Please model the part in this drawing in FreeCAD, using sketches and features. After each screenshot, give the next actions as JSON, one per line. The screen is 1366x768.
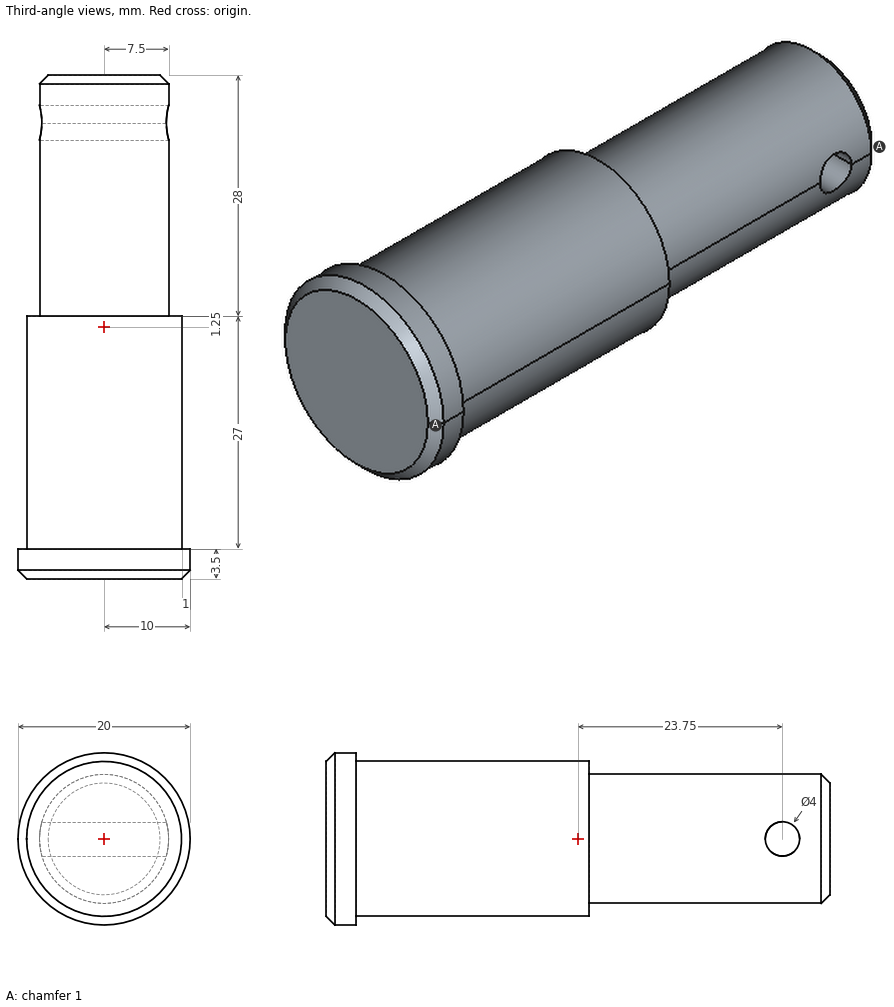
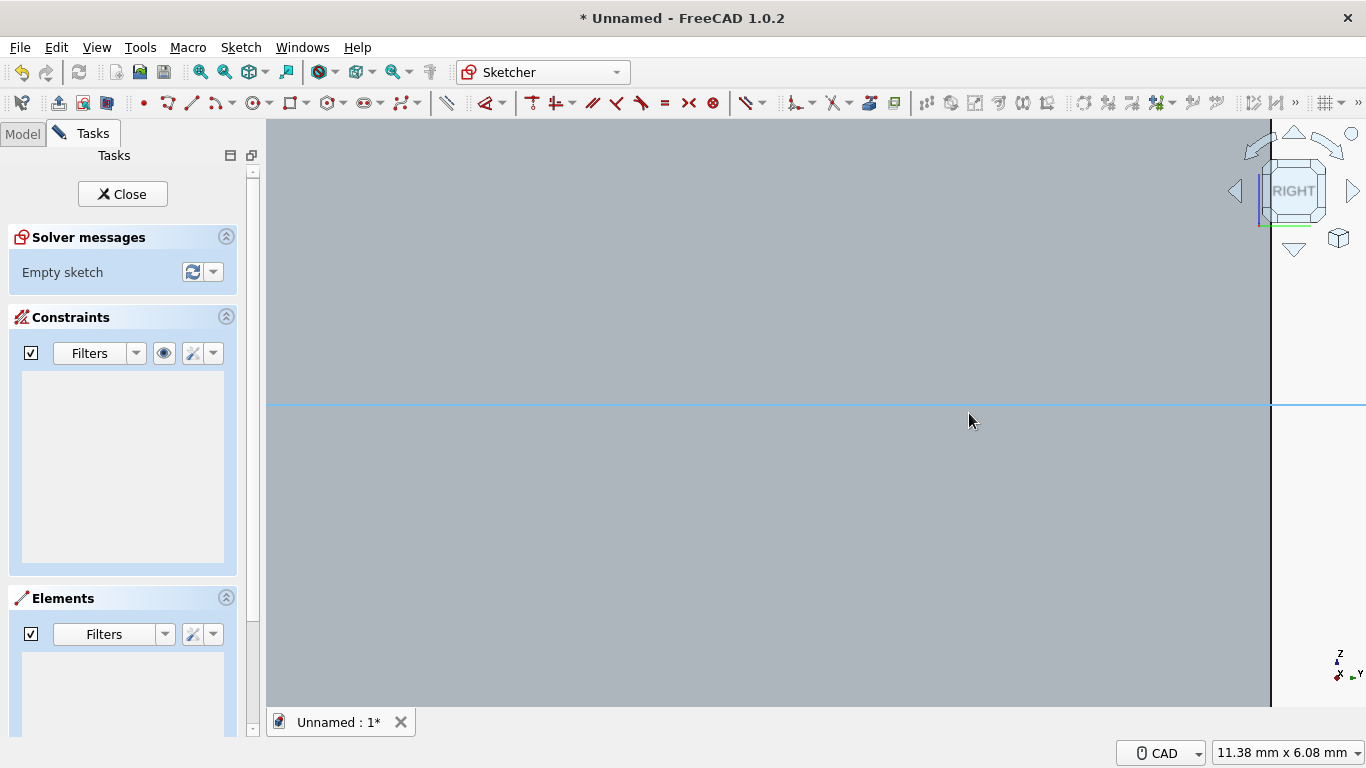
{"action": "left_click", "coordinate": [254, 104]}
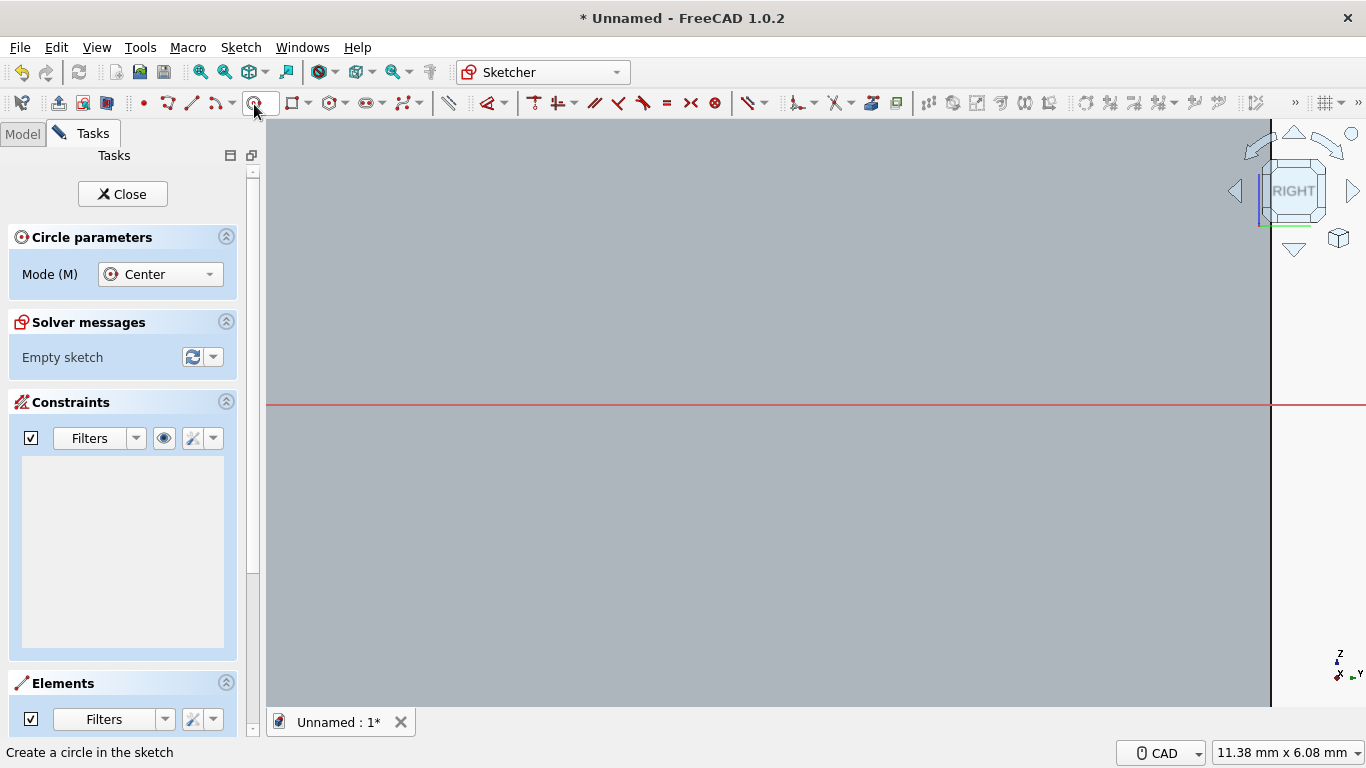
{"action": "left_click", "coordinate": [740, 405]}
{"action": "mouse_move", "coordinate": [876, 269]}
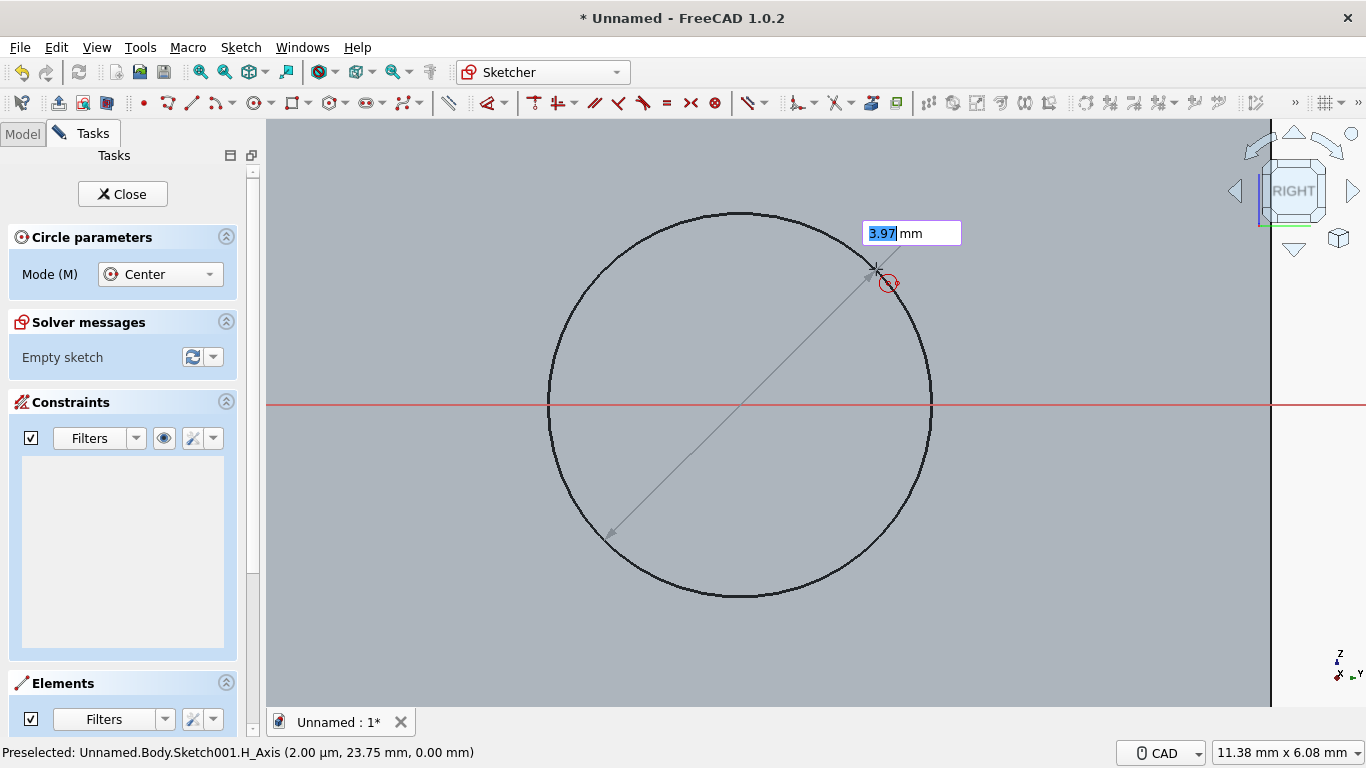
{"action": "type", "text": "4"}
{"action": "key", "text": "Return"}
{"action": "key", "text": "Escape"}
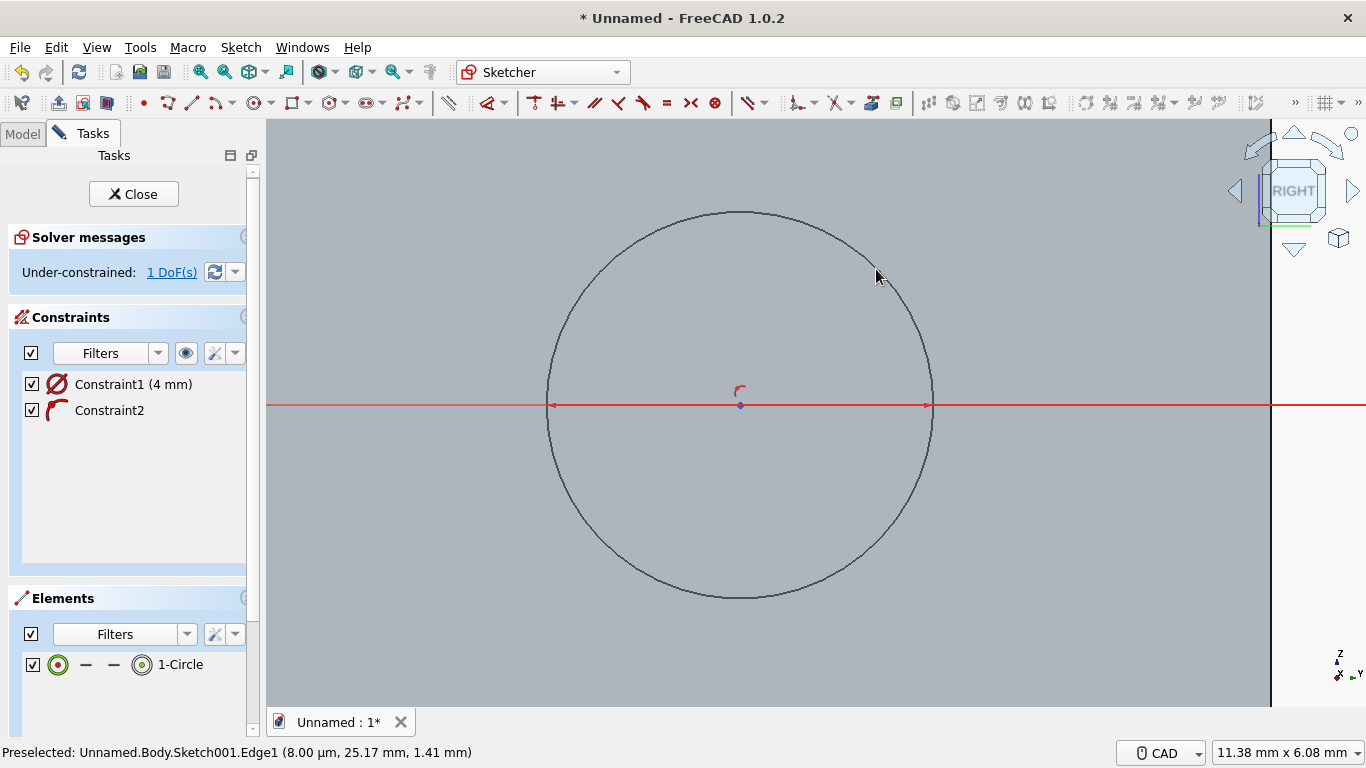
{"action": "left_click", "coordinate": [488, 104]}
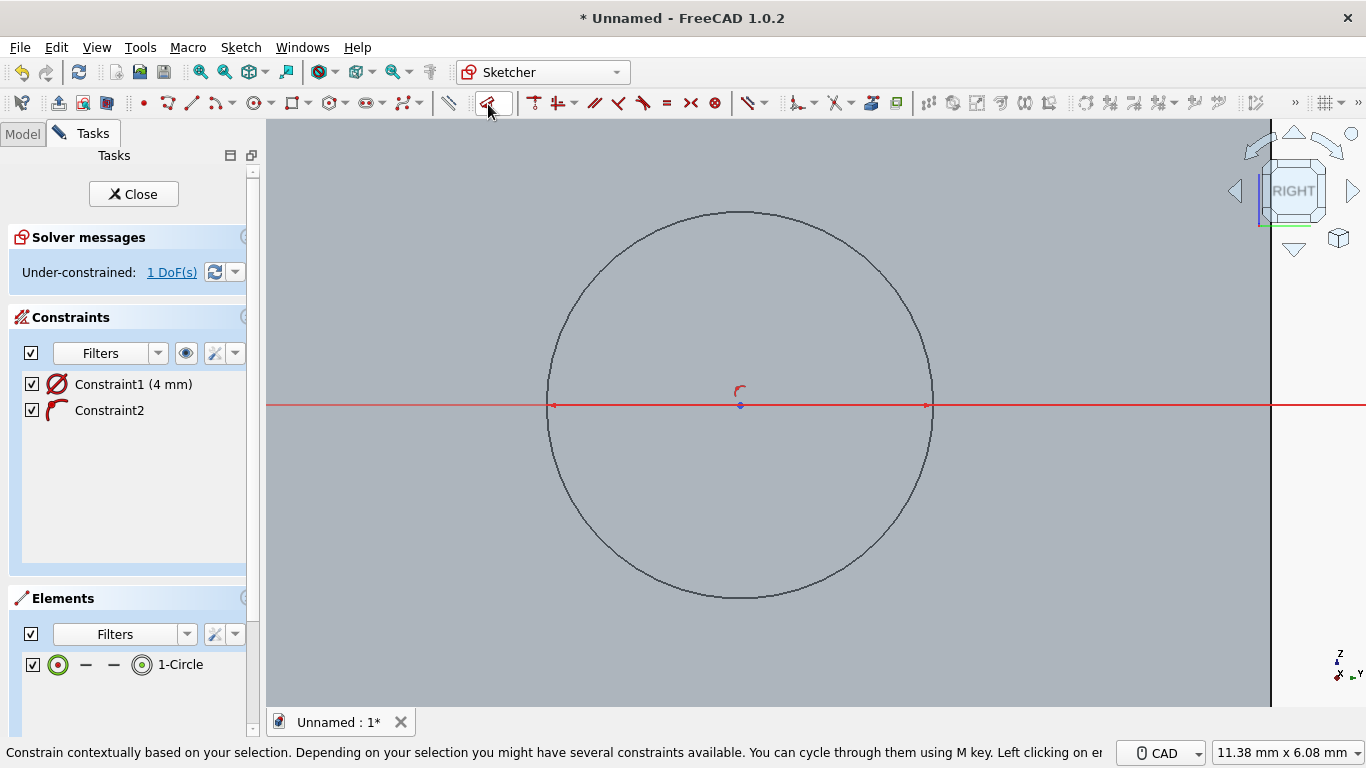
{"action": "left_click", "coordinate": [740, 405]}
{"action": "left_click", "coordinate": [517, 439]}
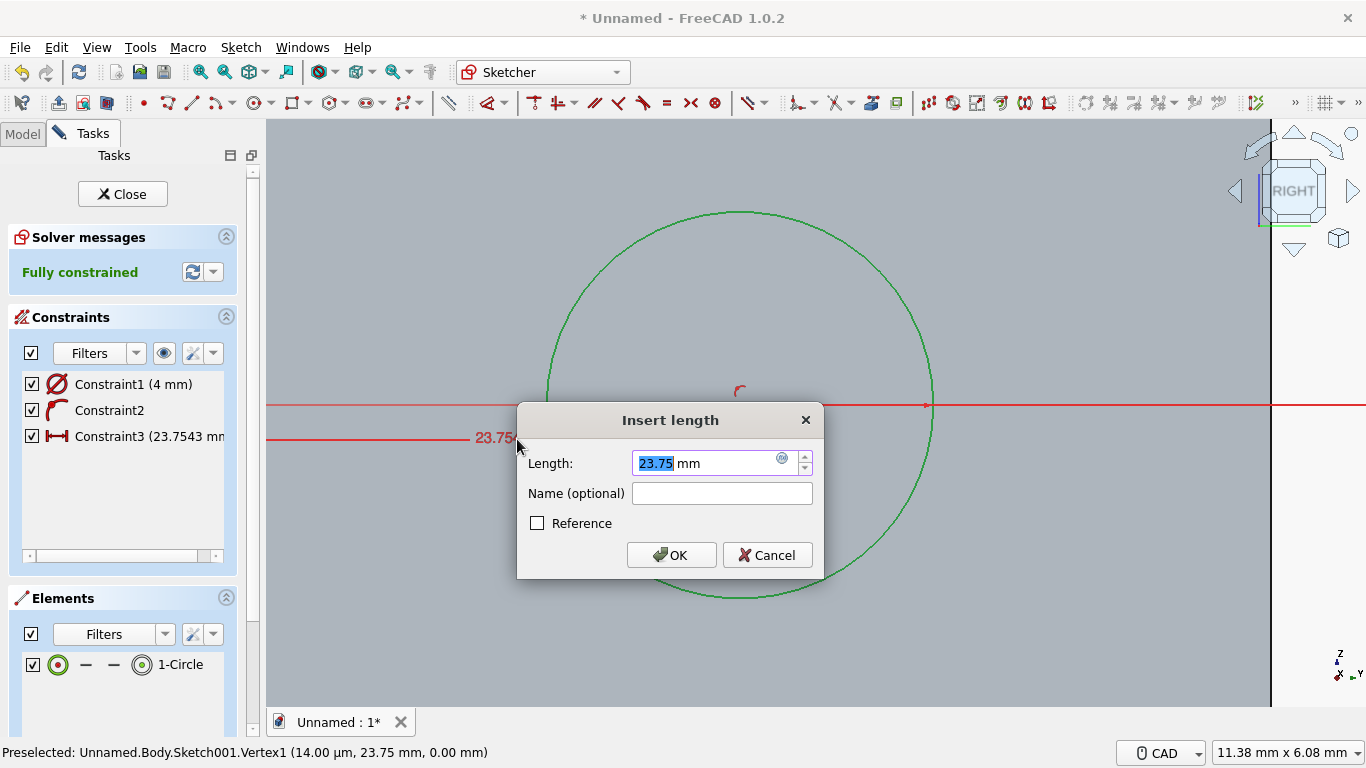
{"action": "type", "text": "23.75"}
{"action": "key", "text": "Return"}
{"action": "key", "text": "Escape"}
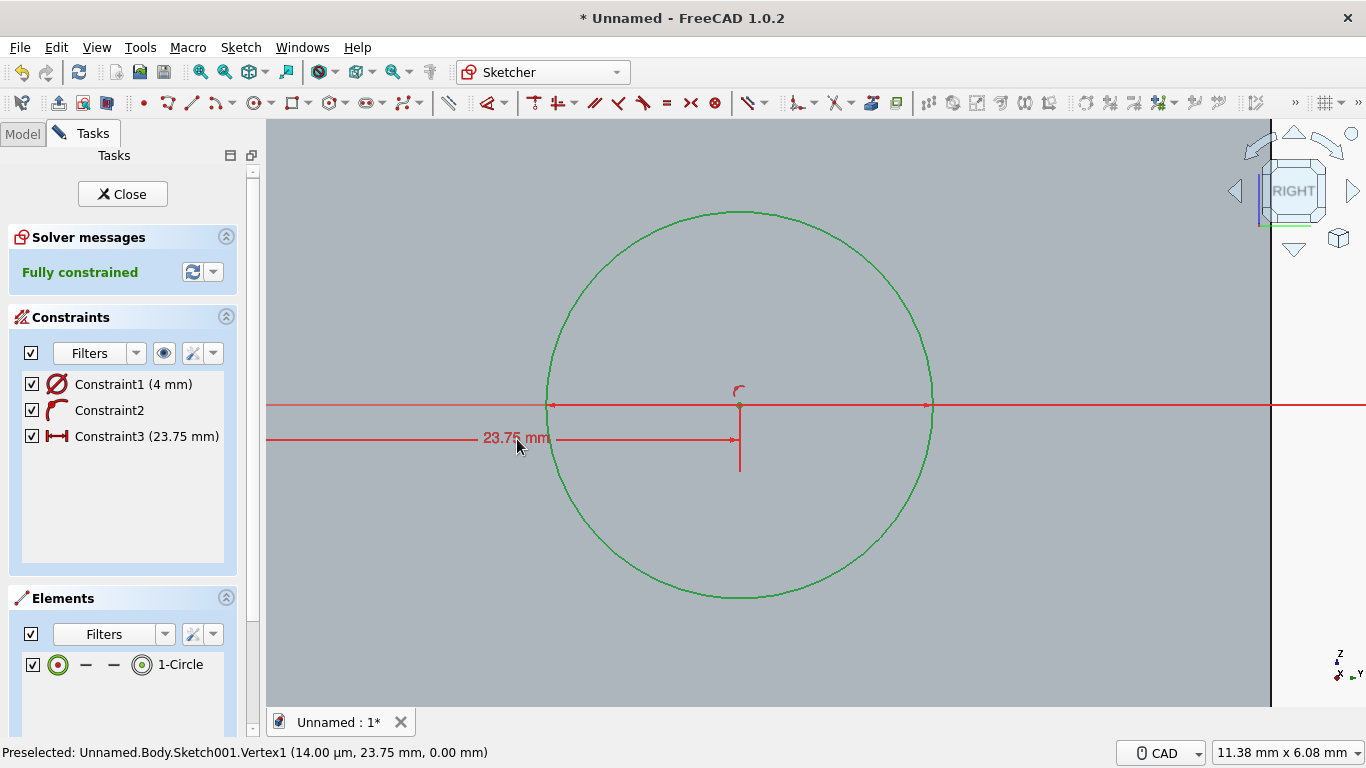
{"action": "left_click", "coordinate": [123, 194]}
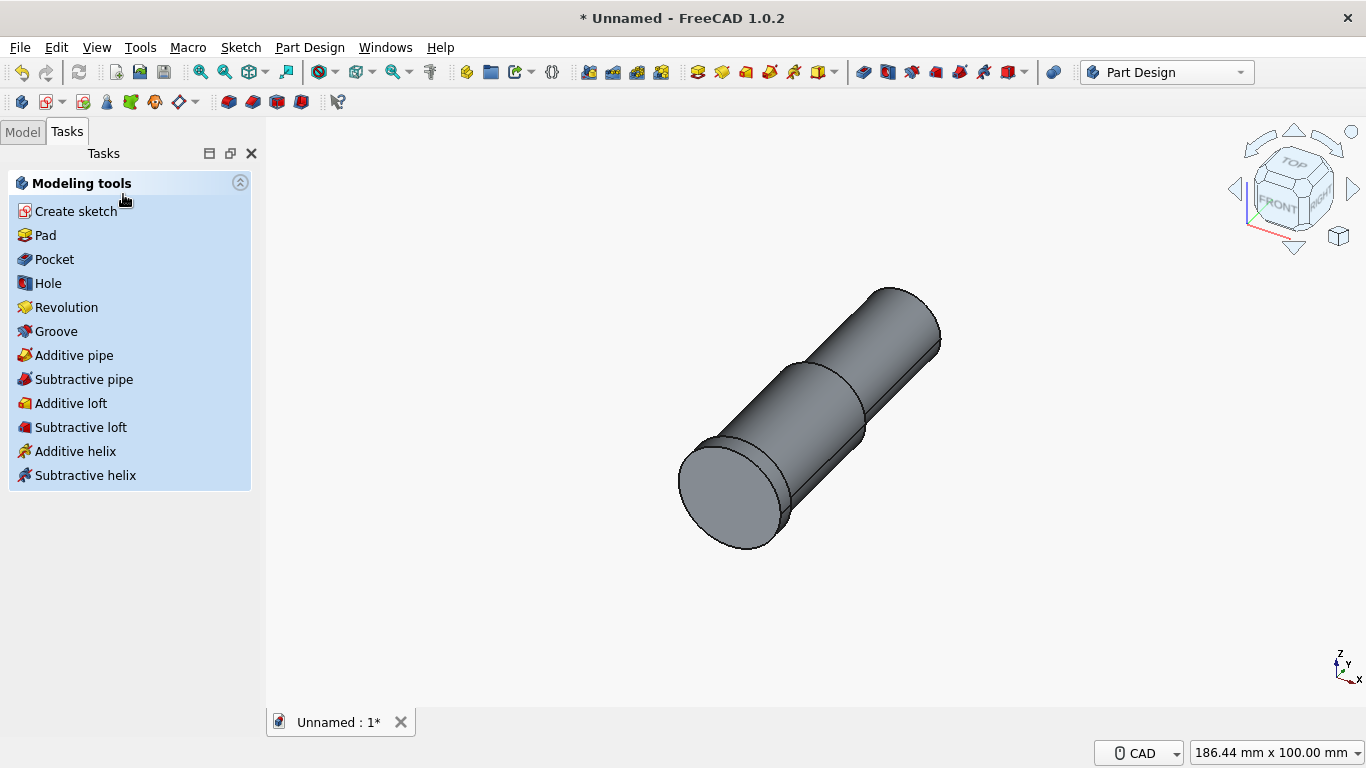
{"action": "left_click", "coordinate": [864, 72]}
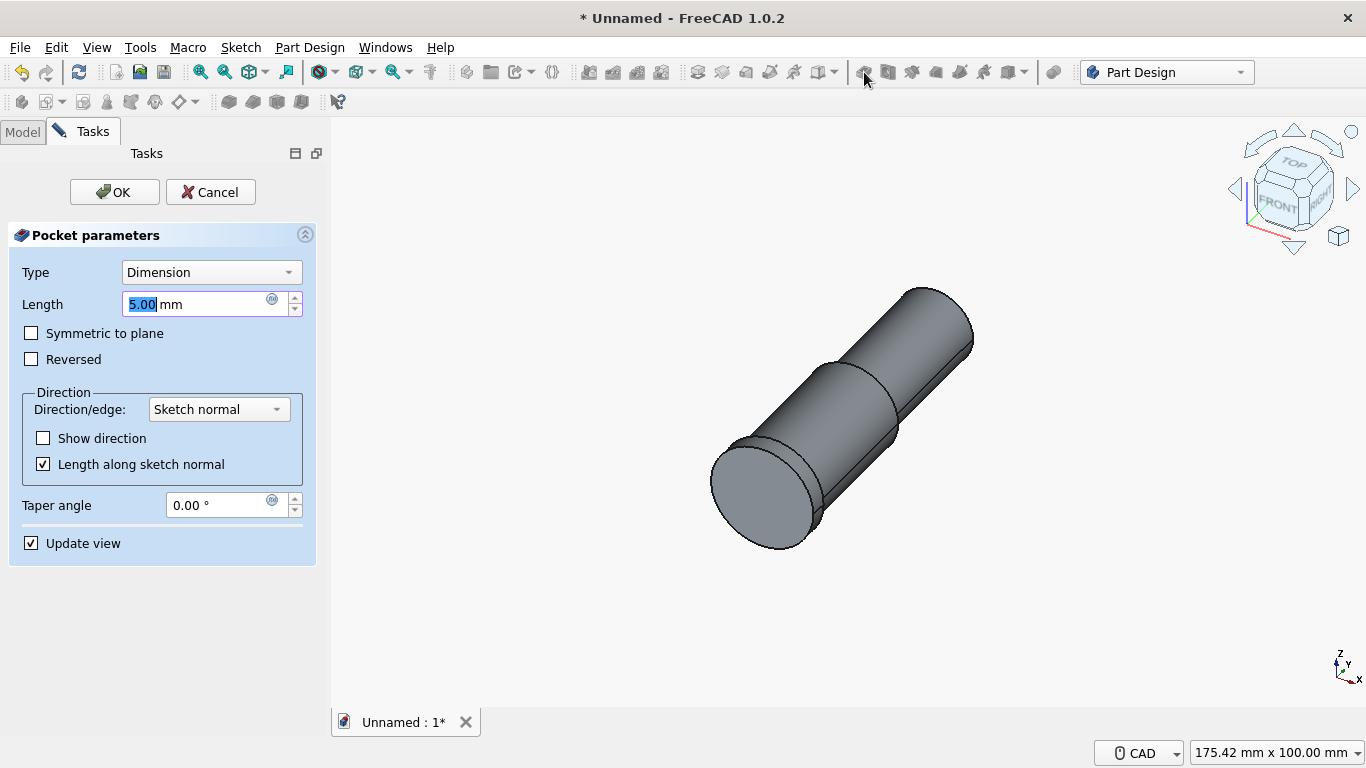
{"action": "type", "text": "20"}
{"action": "key", "text": "Tab"}